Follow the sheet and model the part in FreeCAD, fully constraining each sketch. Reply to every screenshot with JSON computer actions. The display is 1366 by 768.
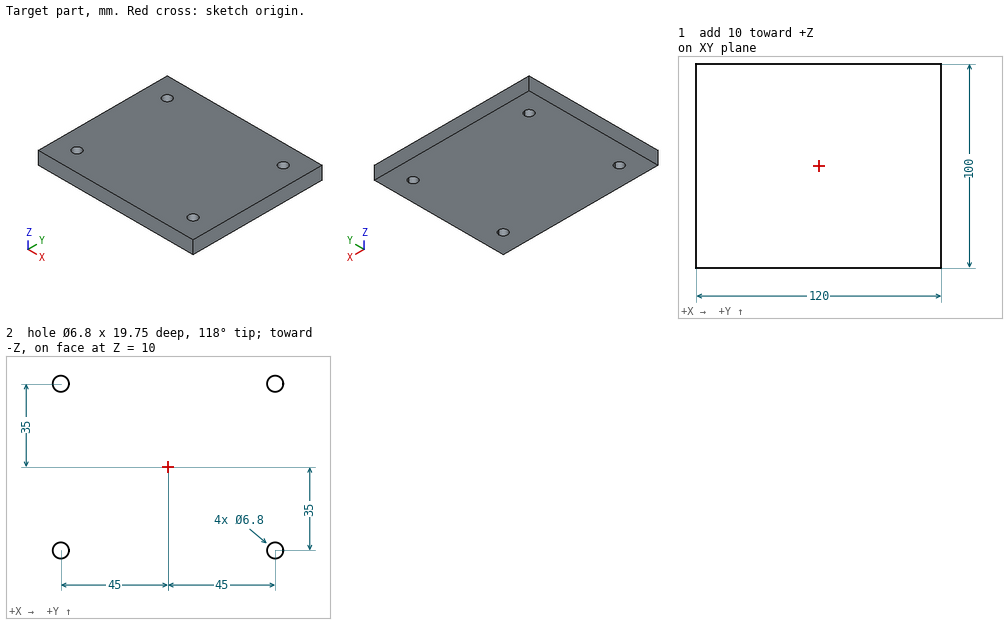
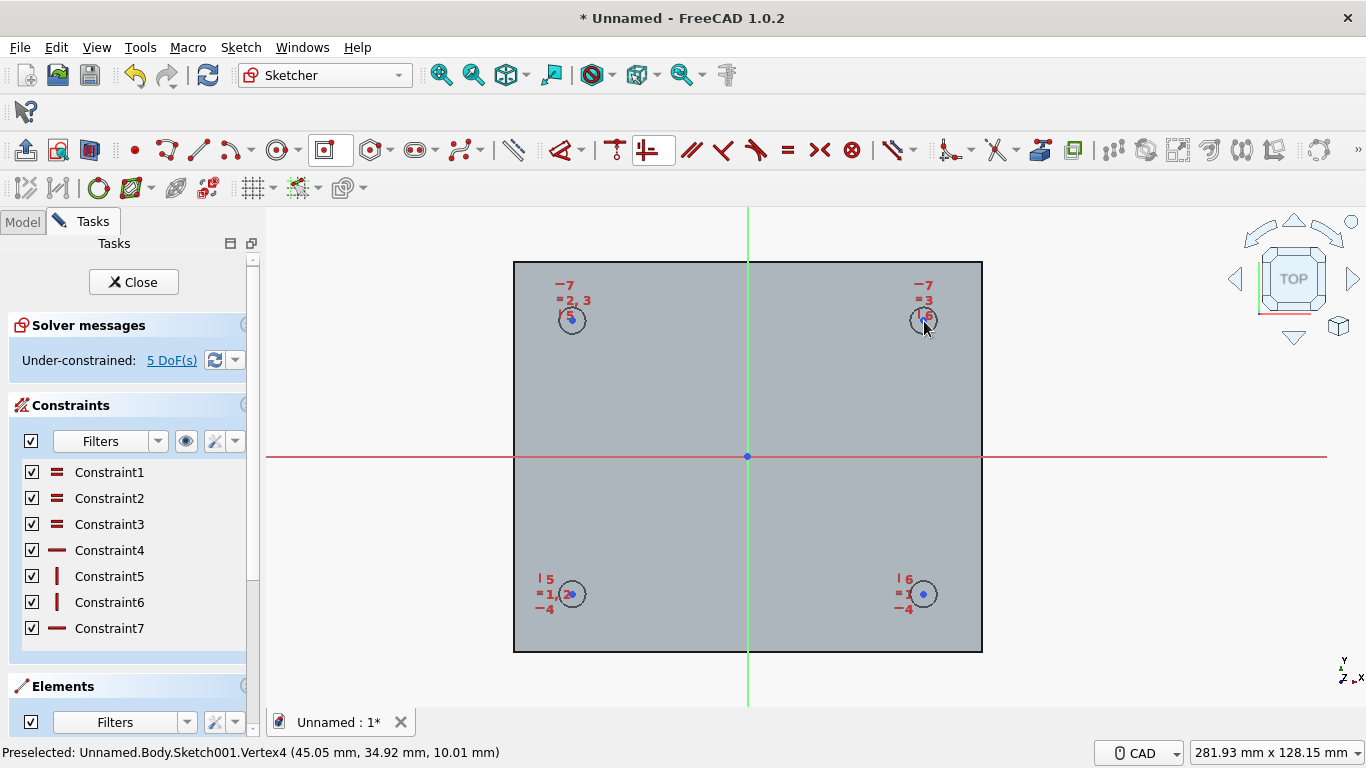
{"action": "left_click", "coordinate": [560, 150]}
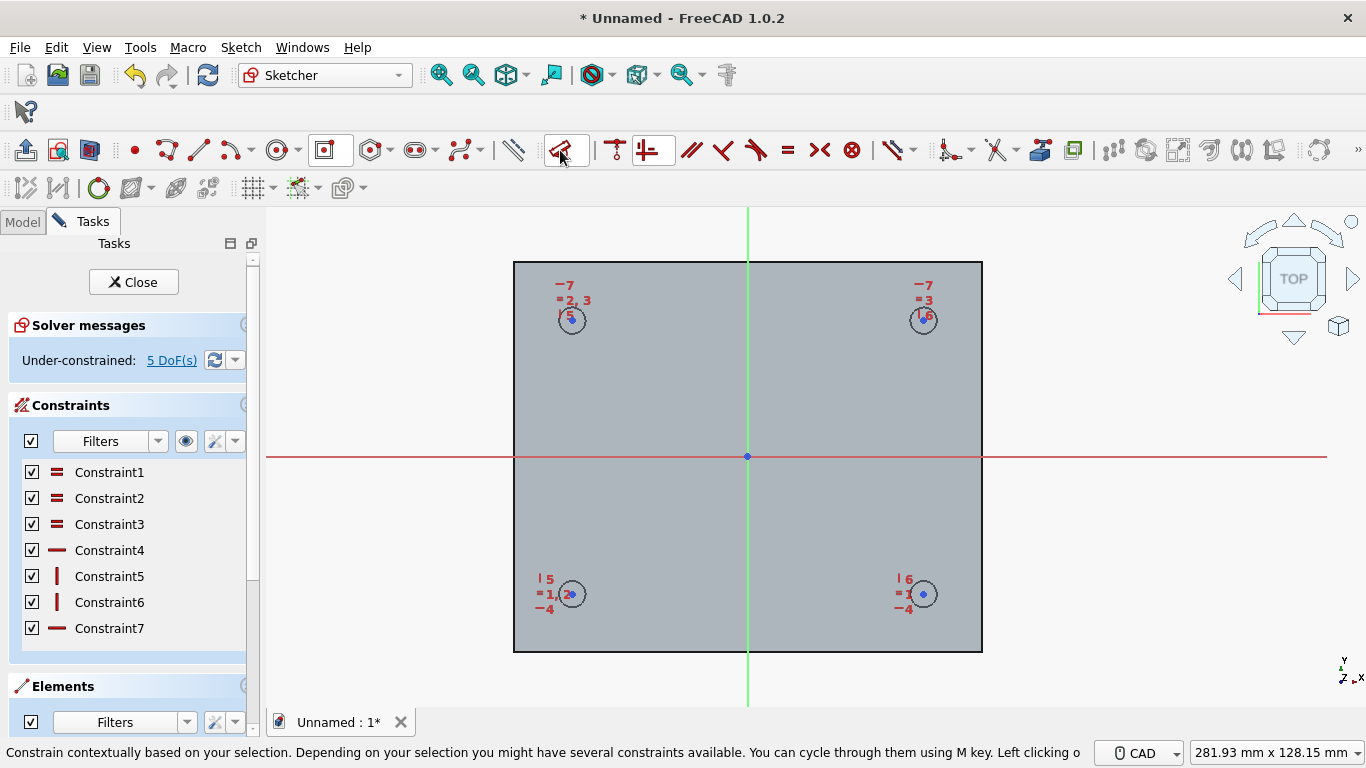
{"action": "scroll", "coordinate": [933, 585], "scroll_direction": "up", "scroll_amount": 3}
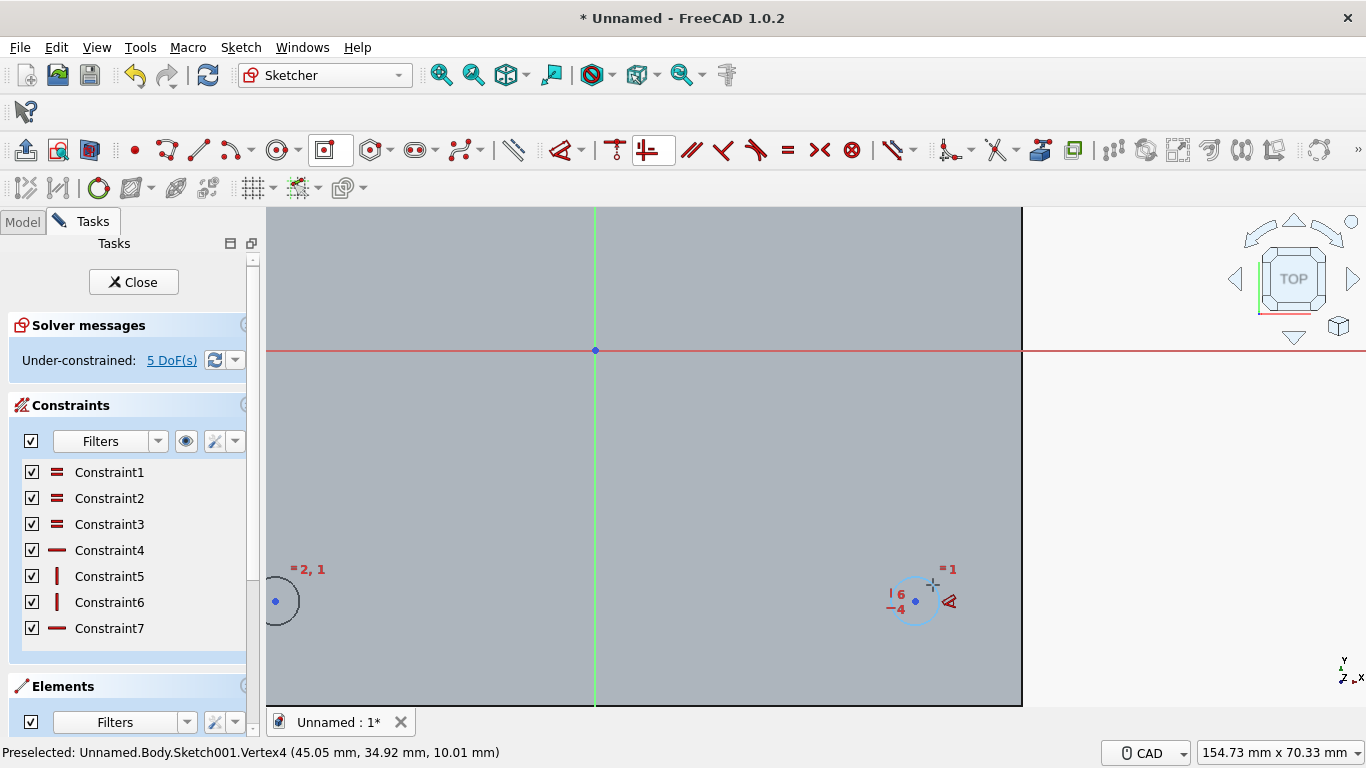
{"action": "left_click", "coordinate": [932, 584]}
{"action": "left_click", "coordinate": [954, 561]}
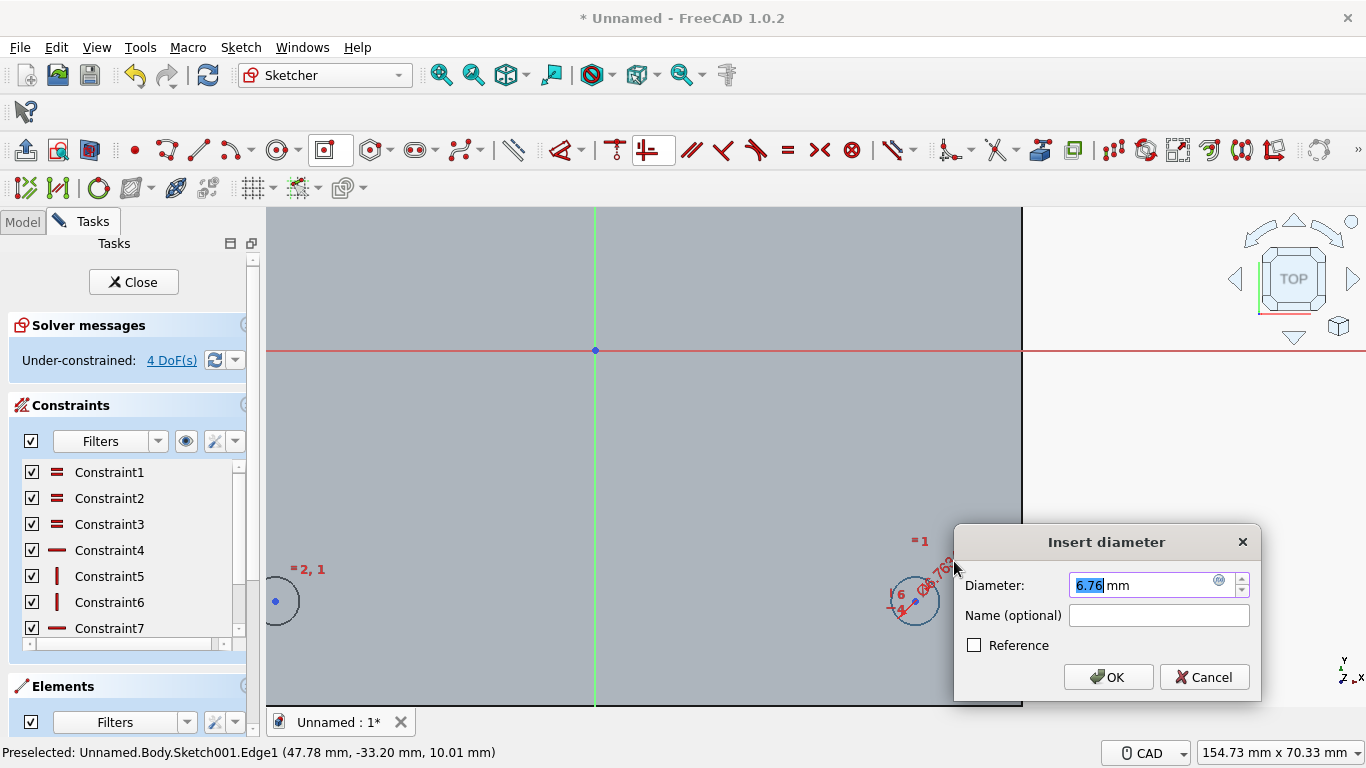
{"action": "type", "text": "6.8"}
{"action": "key", "text": "Return"}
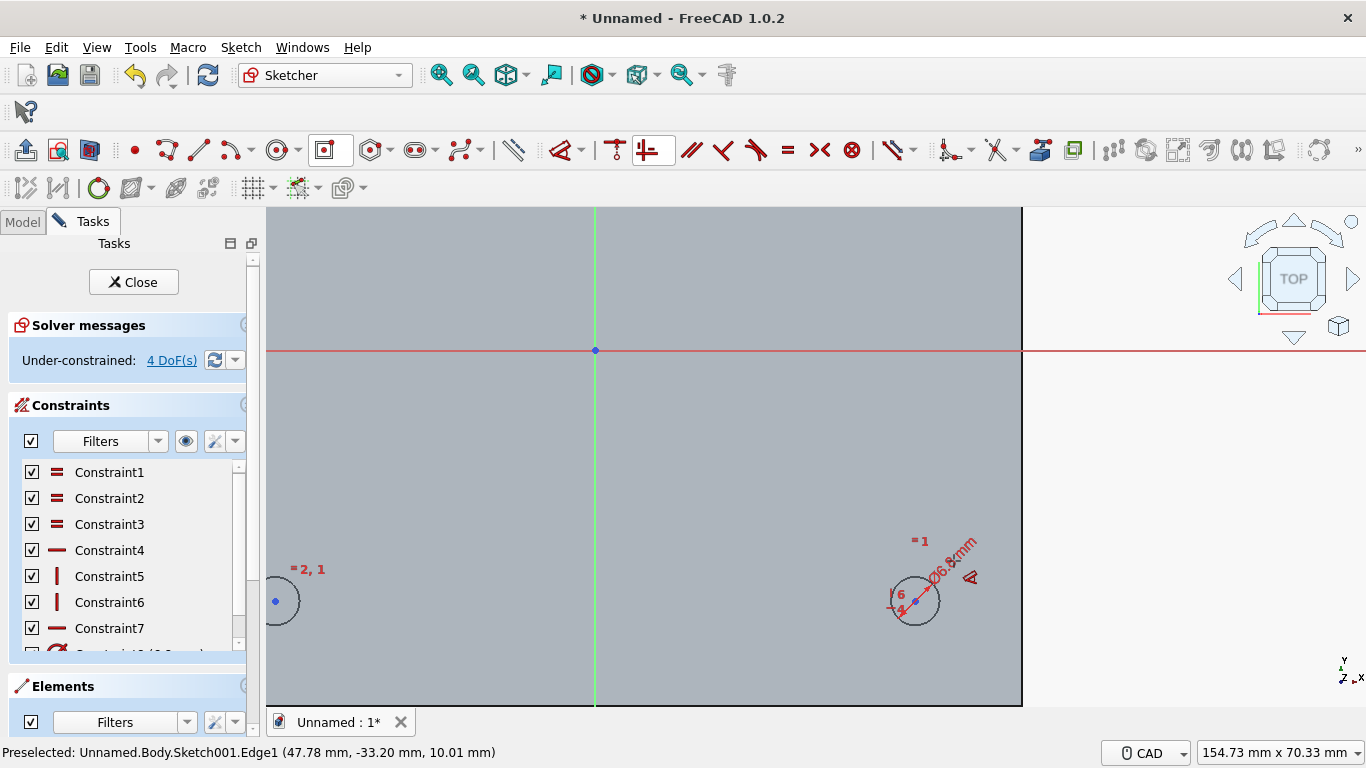
{"action": "left_click", "coordinate": [915, 601]}
{"action": "left_click", "coordinate": [755, 635]}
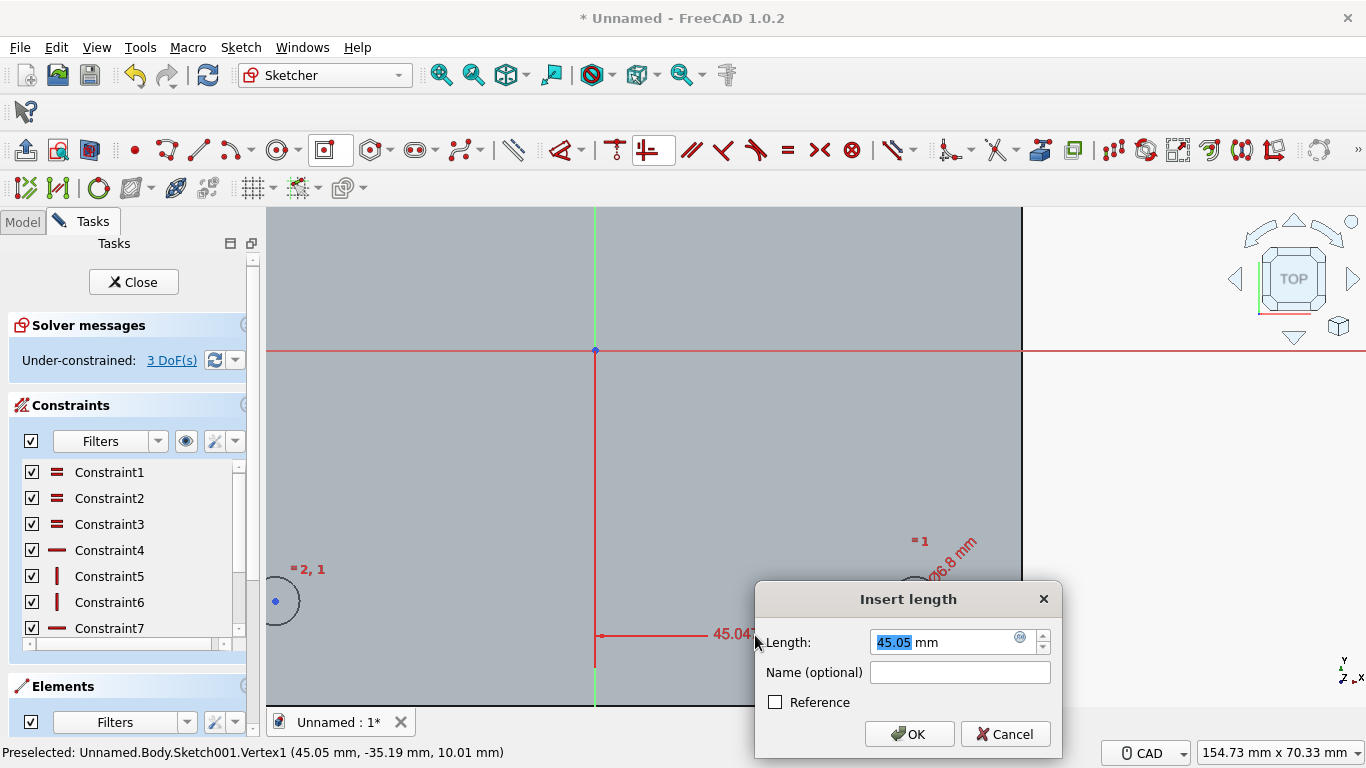
{"action": "type", "text": "45"}
{"action": "key", "text": "Return"}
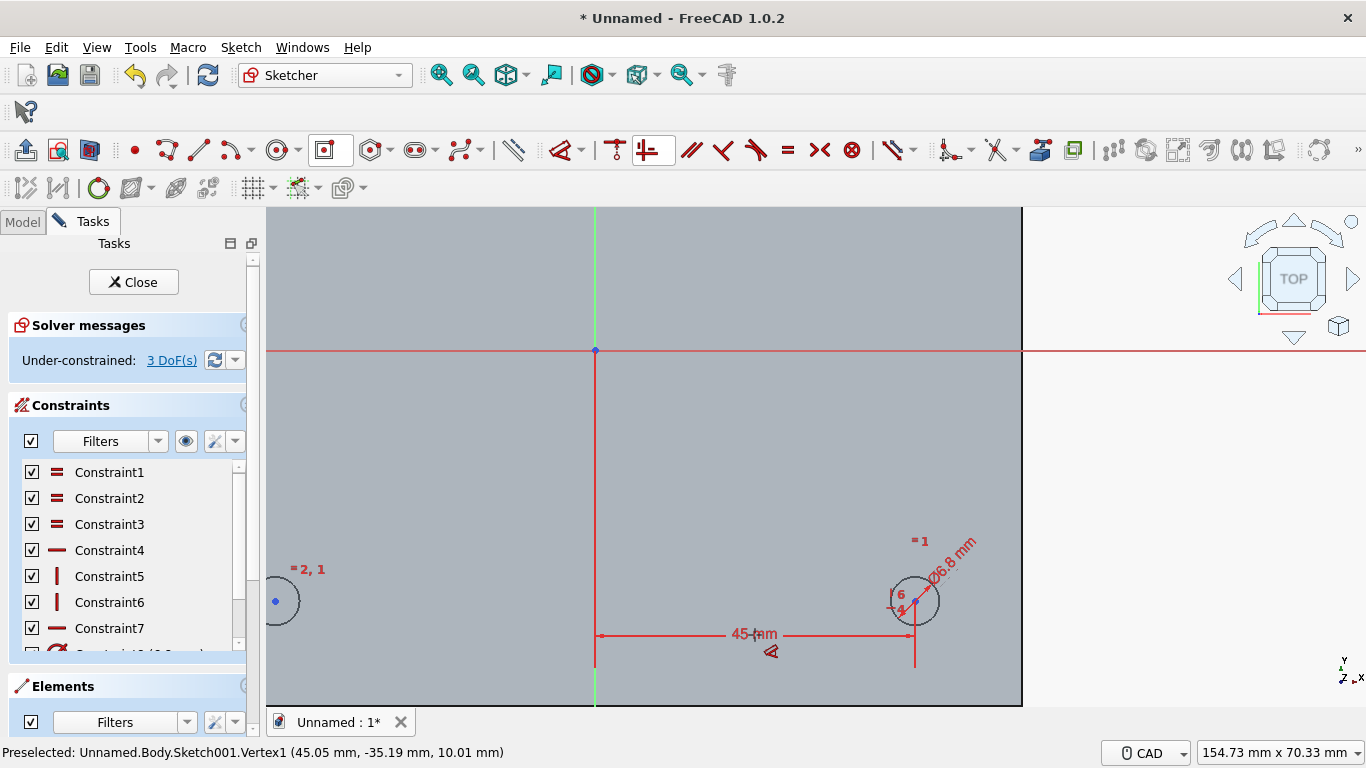
{"action": "left_click", "coordinate": [915, 601]}
{"action": "left_click", "coordinate": [949, 476]}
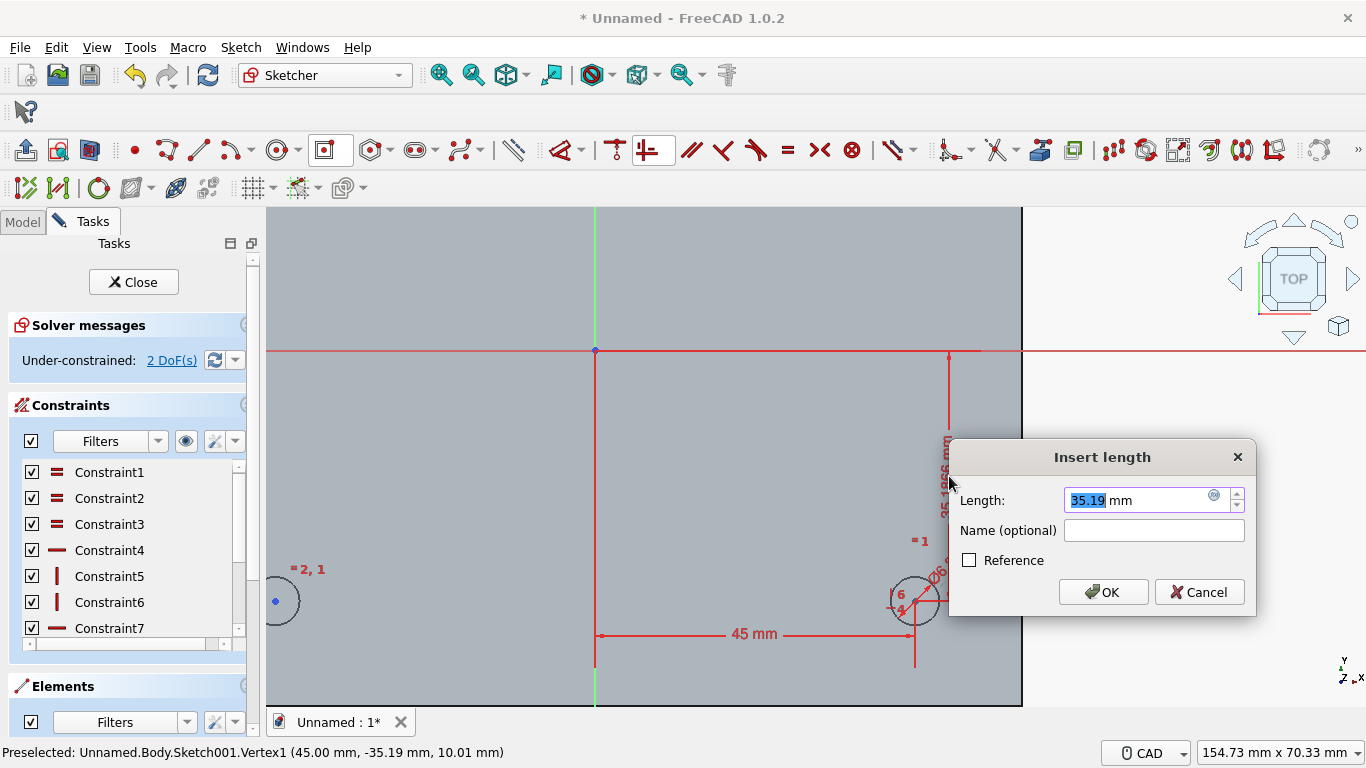
{"action": "type", "text": "35"}
{"action": "key", "text": "Return"}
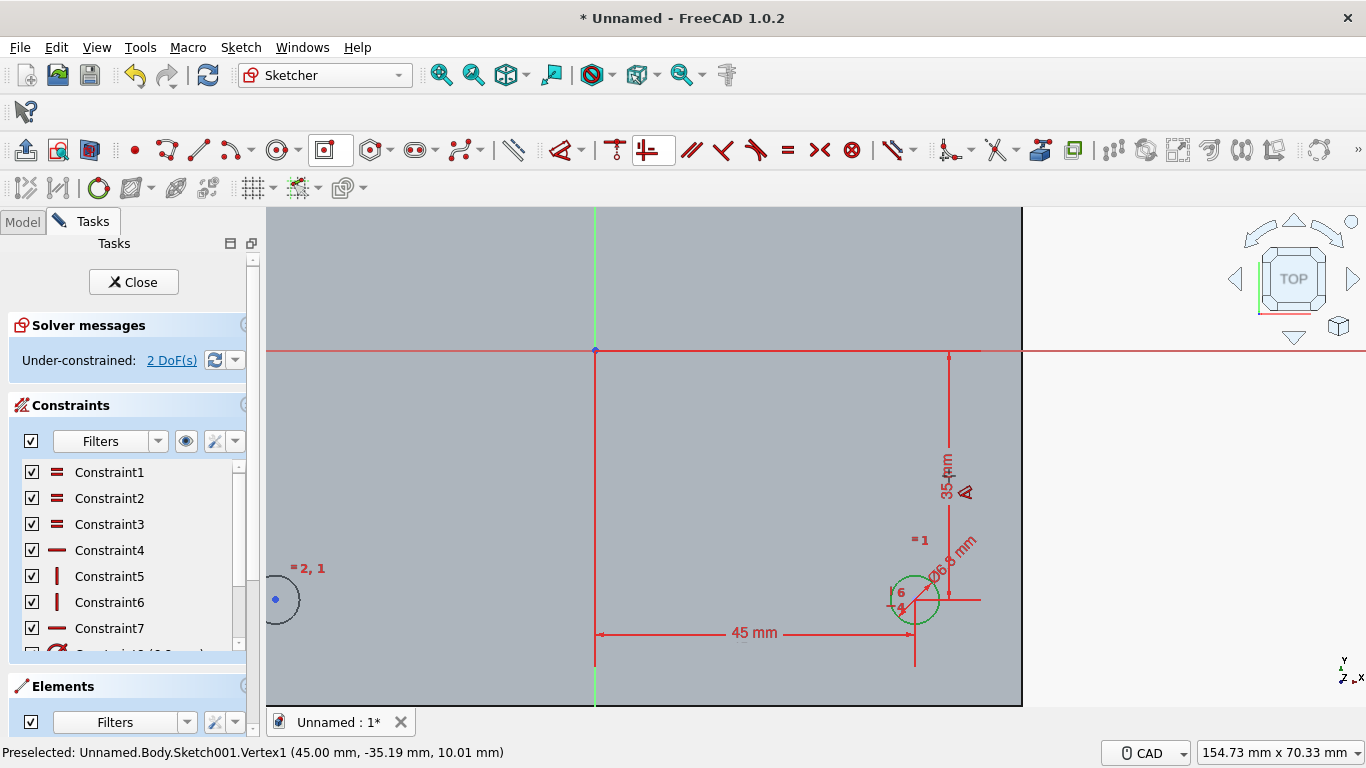
{"action": "scroll", "coordinate": [933, 586], "scroll_direction": "down", "scroll_amount": 3}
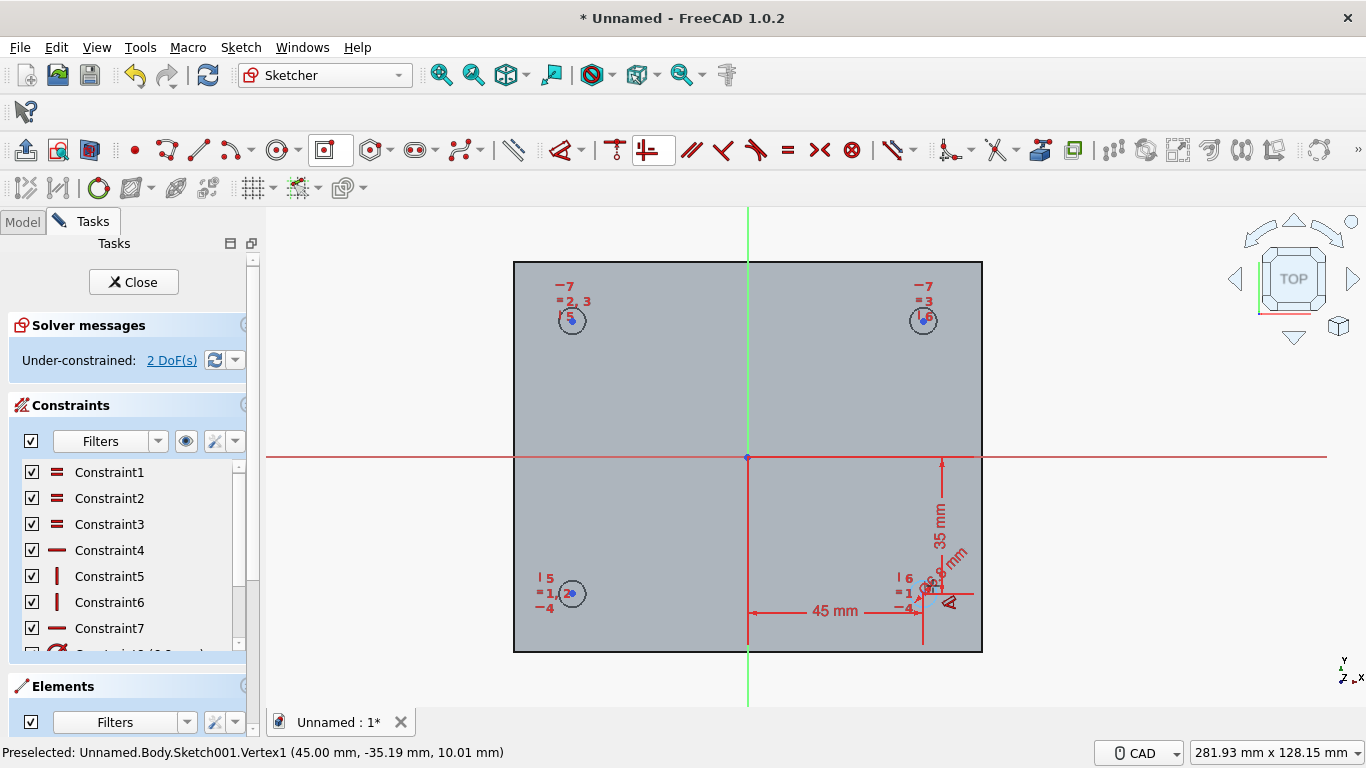
{"action": "left_click", "coordinate": [572, 594]}
{"action": "left_click", "coordinate": [660, 628]}